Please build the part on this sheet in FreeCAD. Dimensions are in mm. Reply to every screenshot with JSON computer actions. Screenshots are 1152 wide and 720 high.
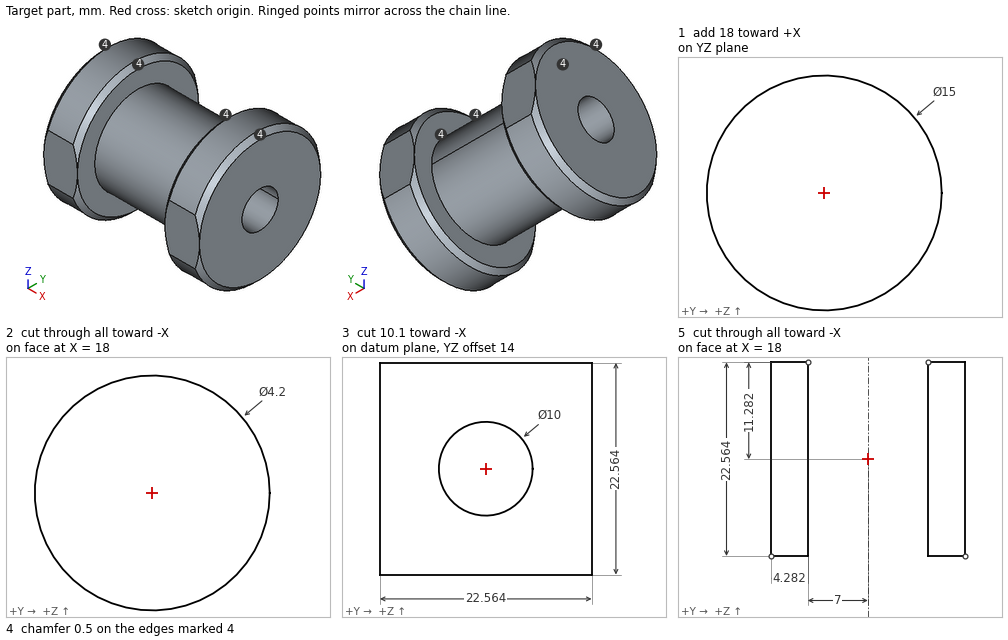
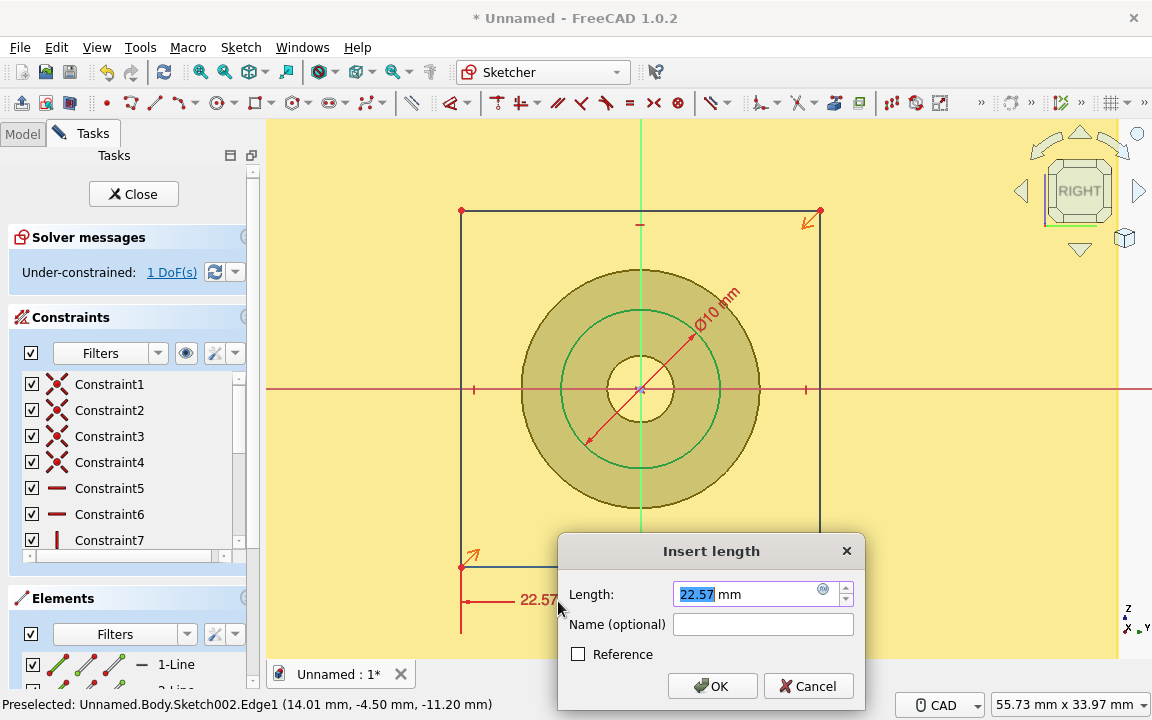
{"action": "type", "text": "22.564"}
{"action": "key", "text": "Return"}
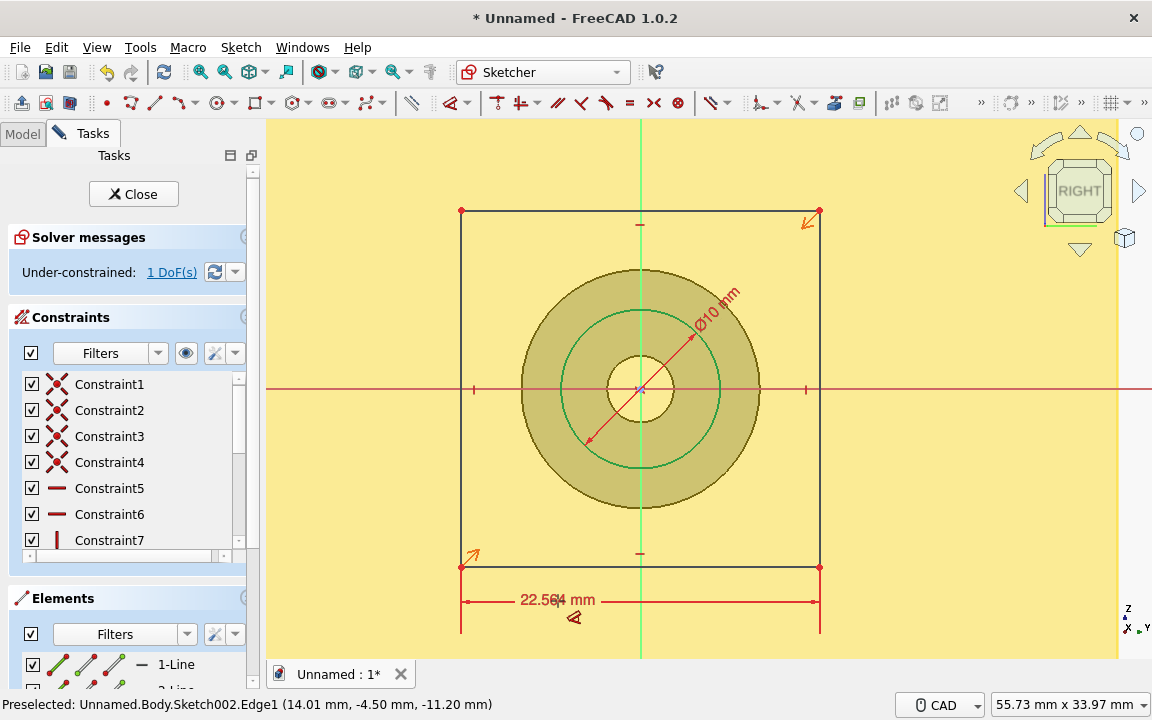
{"action": "left_click", "coordinate": [820, 460]}
{"action": "left_click", "coordinate": [854, 307]}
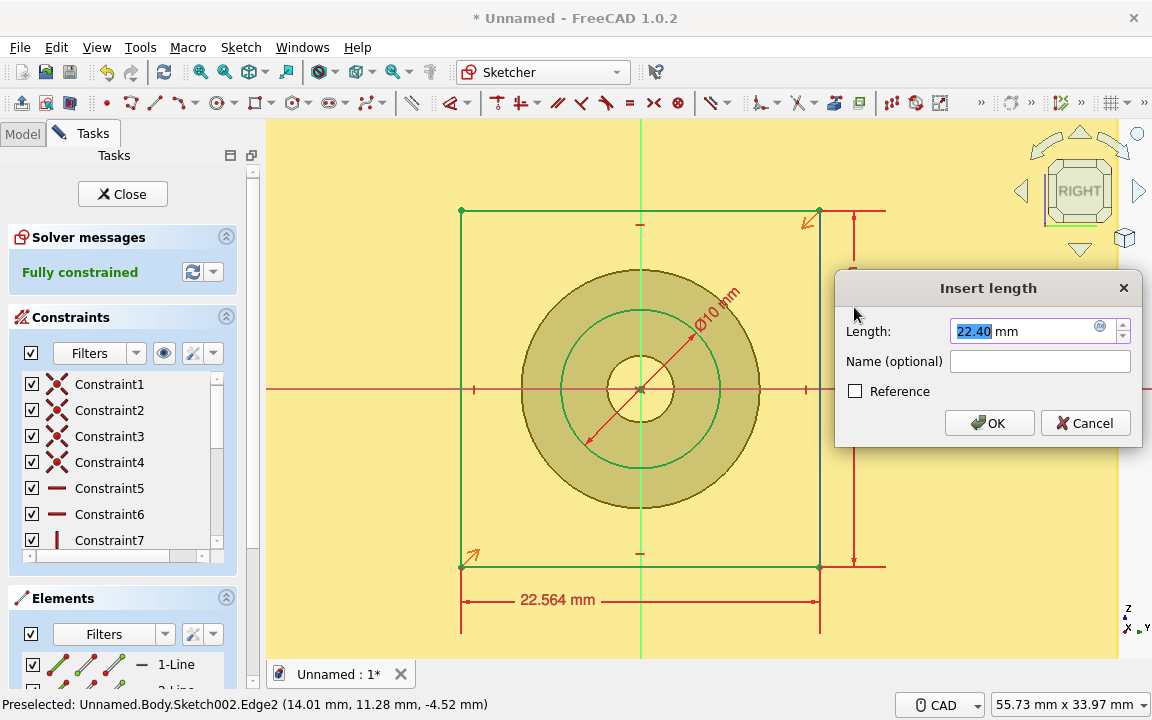
{"action": "type", "text": "22.564"}
{"action": "key", "text": "Return"}
{"action": "key", "text": "Escape"}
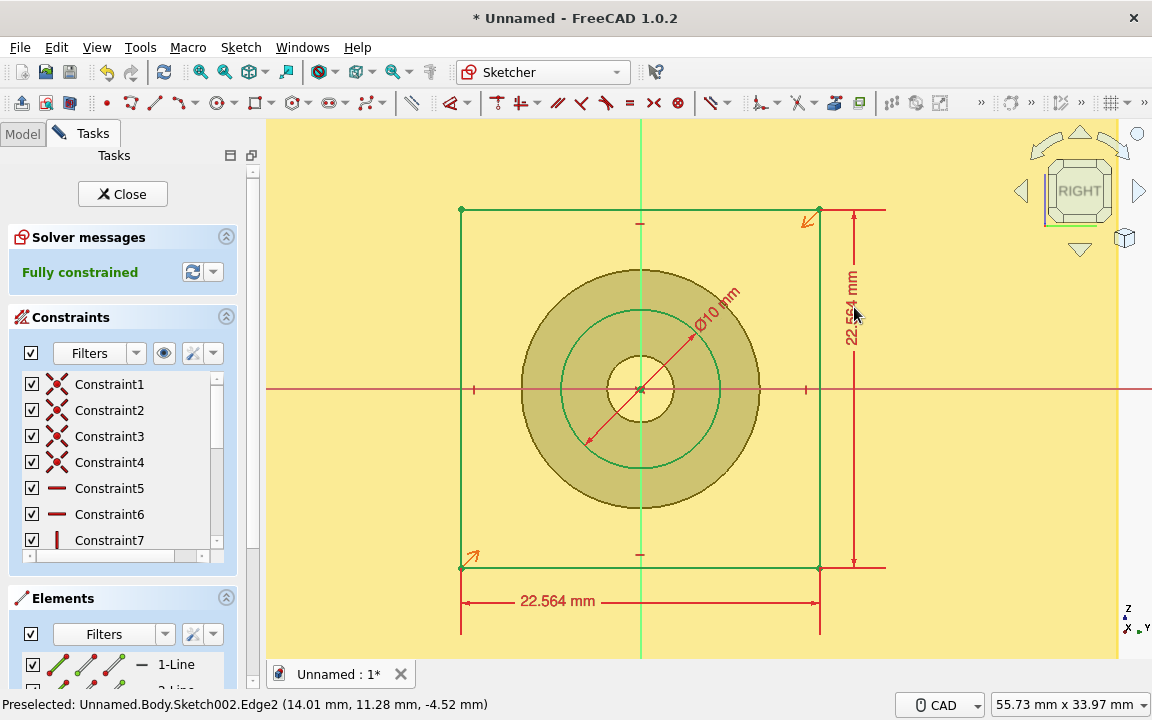
{"action": "left_click", "coordinate": [123, 194]}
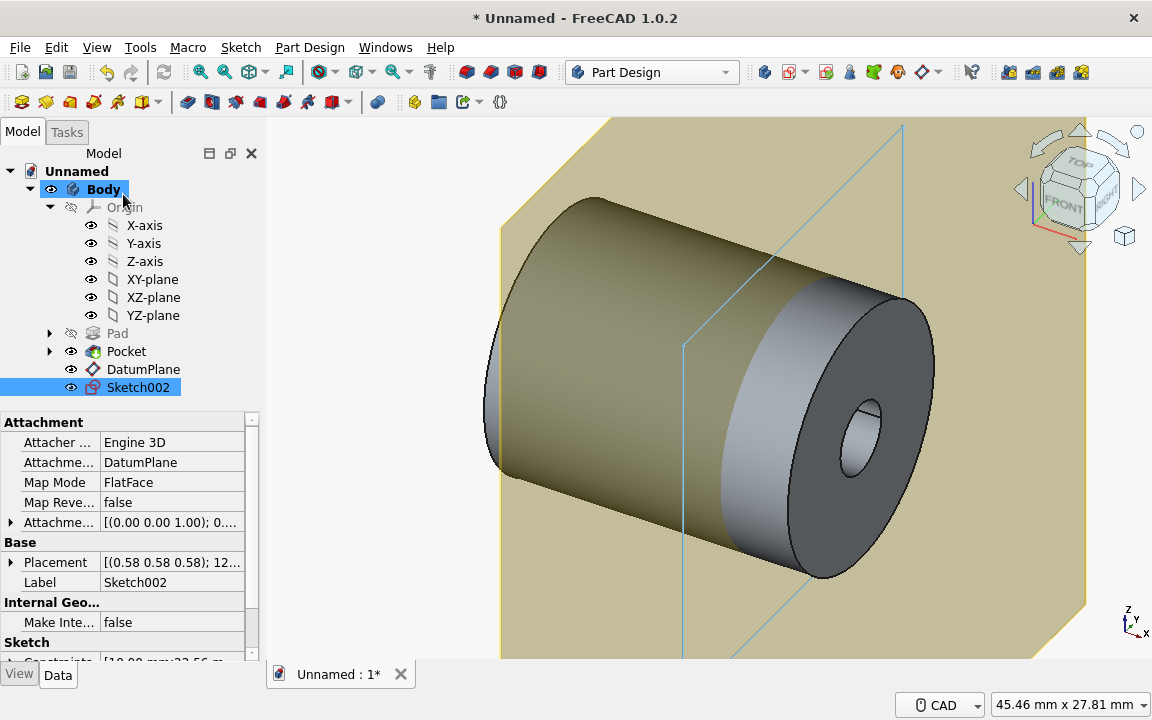
{"action": "left_click", "coordinate": [188, 102]}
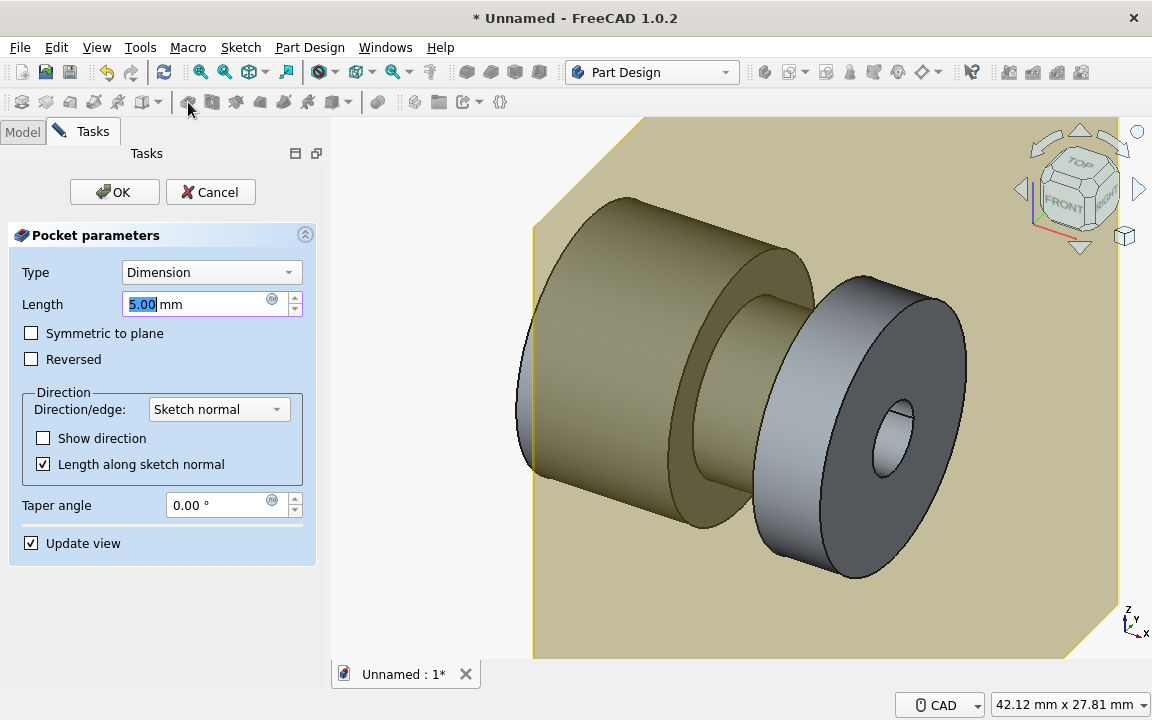
{"action": "type", "text": "10.1"}
{"action": "key", "text": "Tab"}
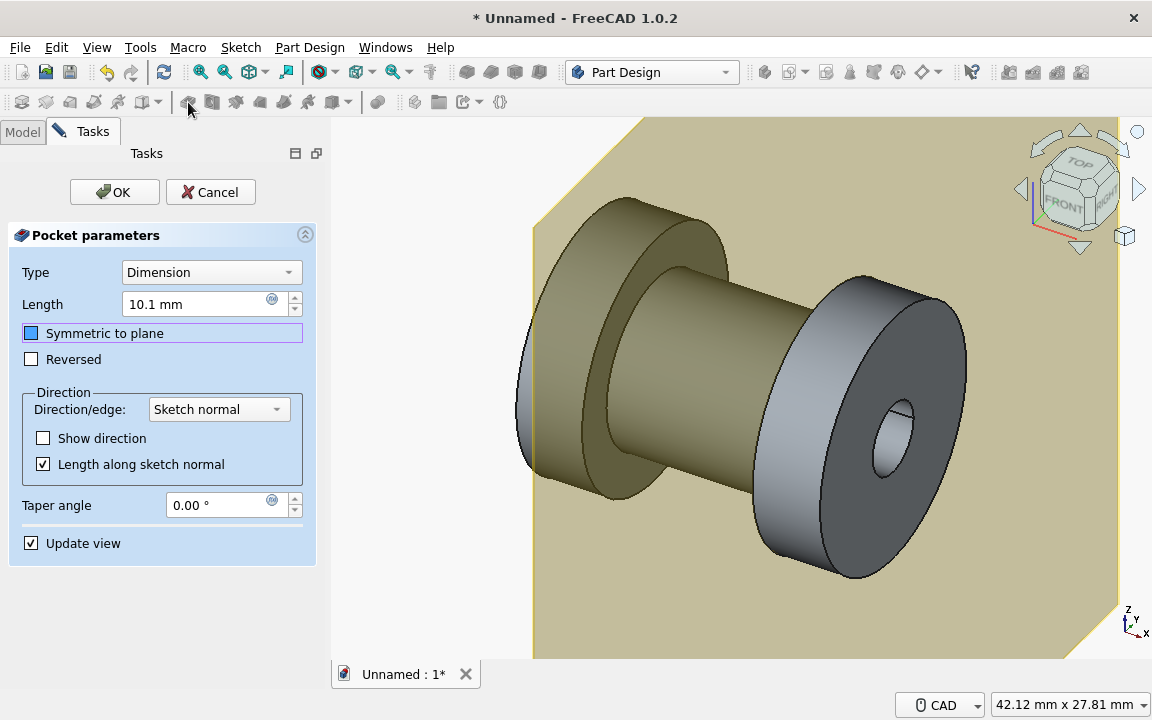
{"action": "left_click", "coordinate": [115, 192]}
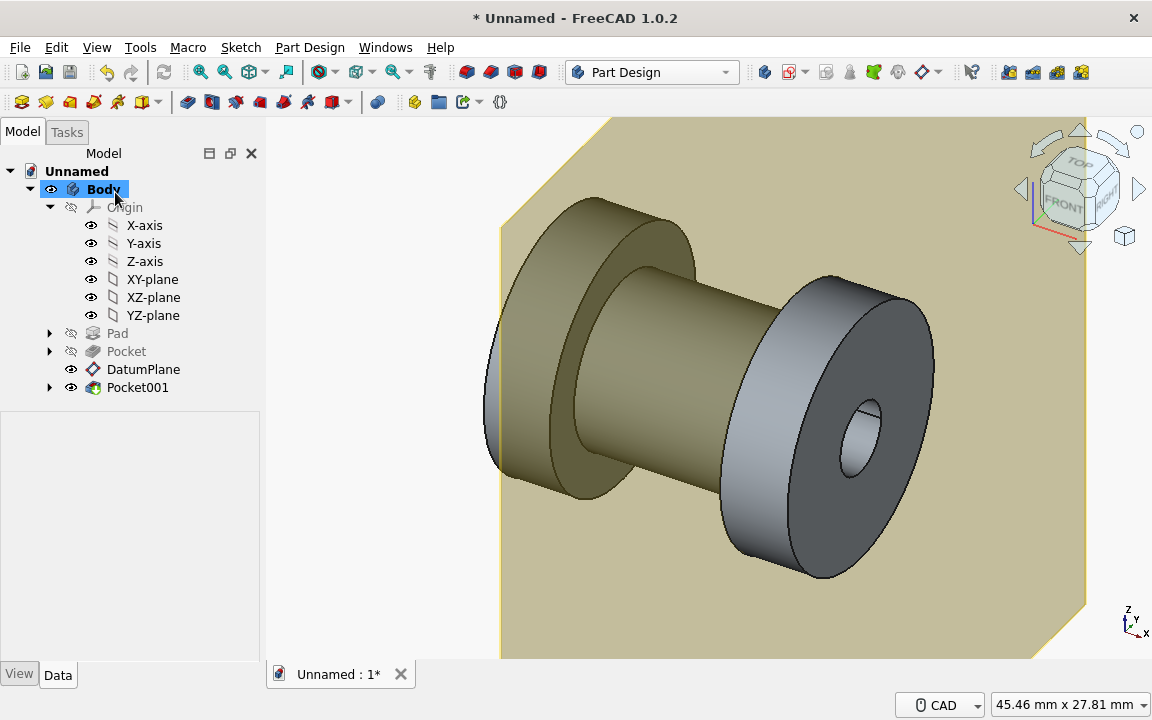
{"action": "left_click", "coordinate": [116, 369]}
{"action": "key", "text": "space"}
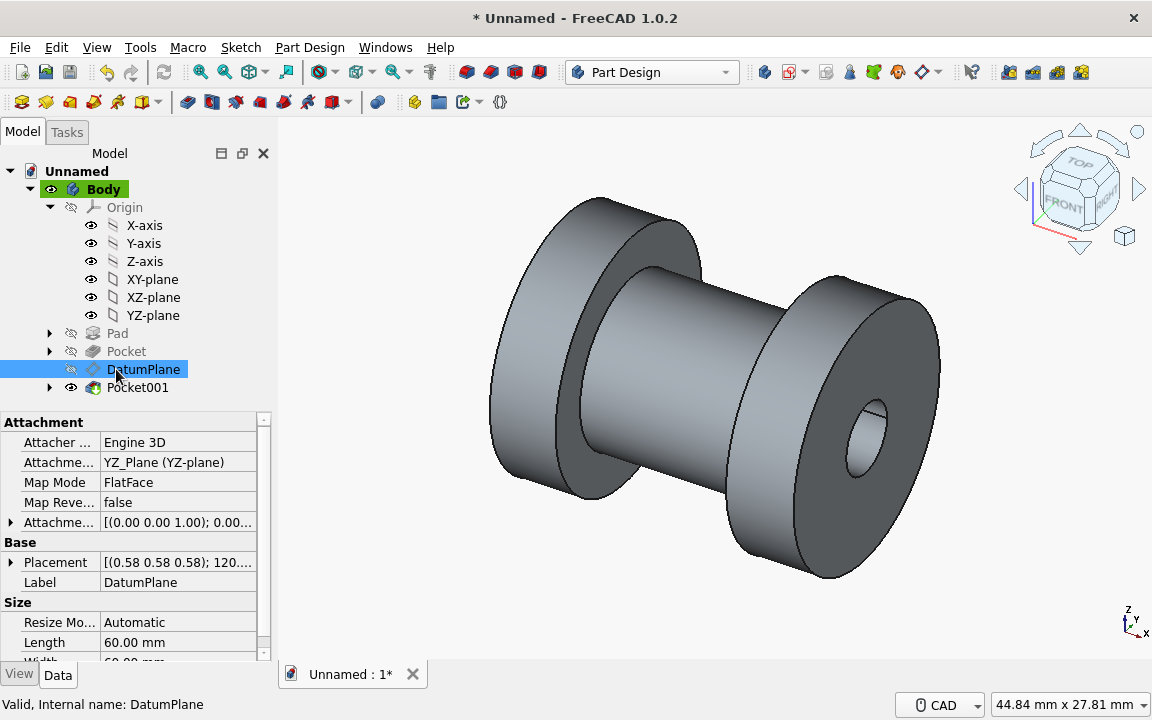
{"action": "left_click", "coordinate": [556, 431]}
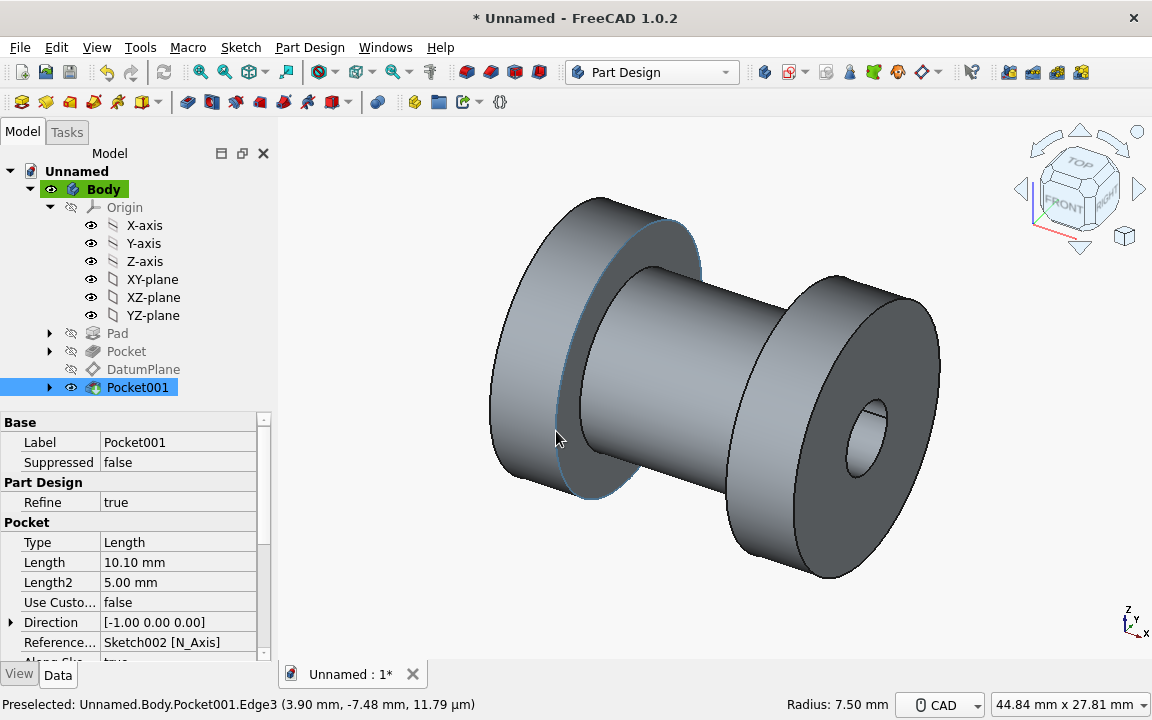
{"action": "left_click", "coordinate": [794, 510], "text": "ctrl"}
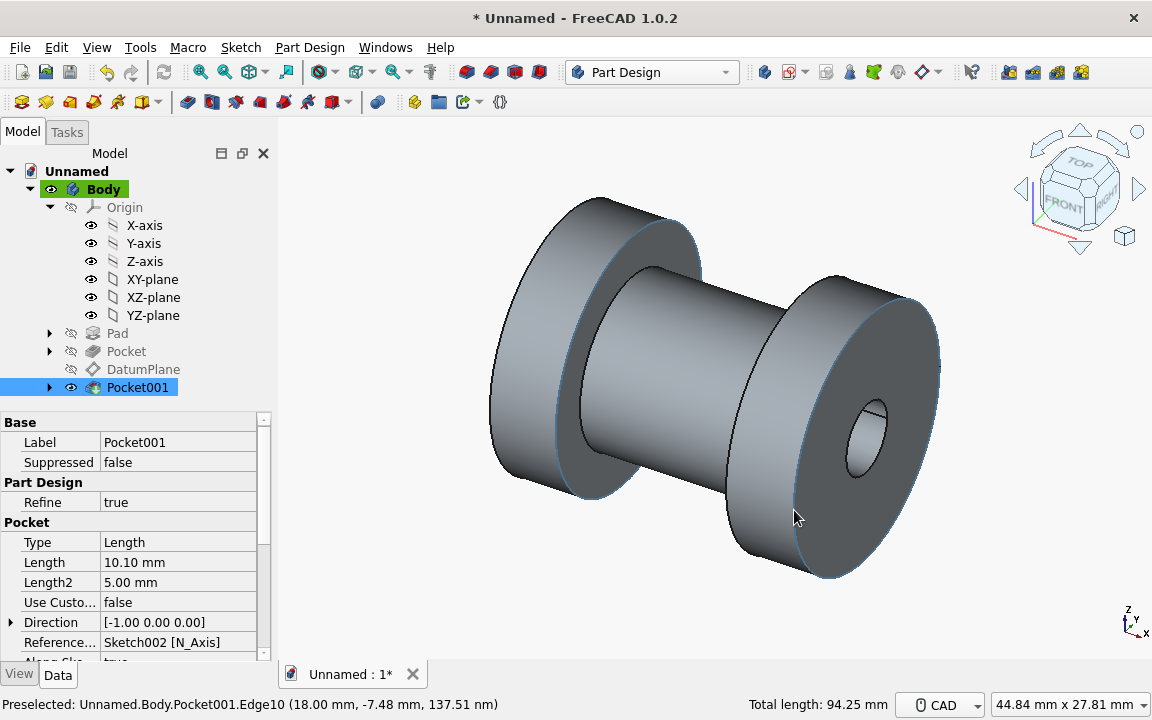
{"action": "key", "text": "0"}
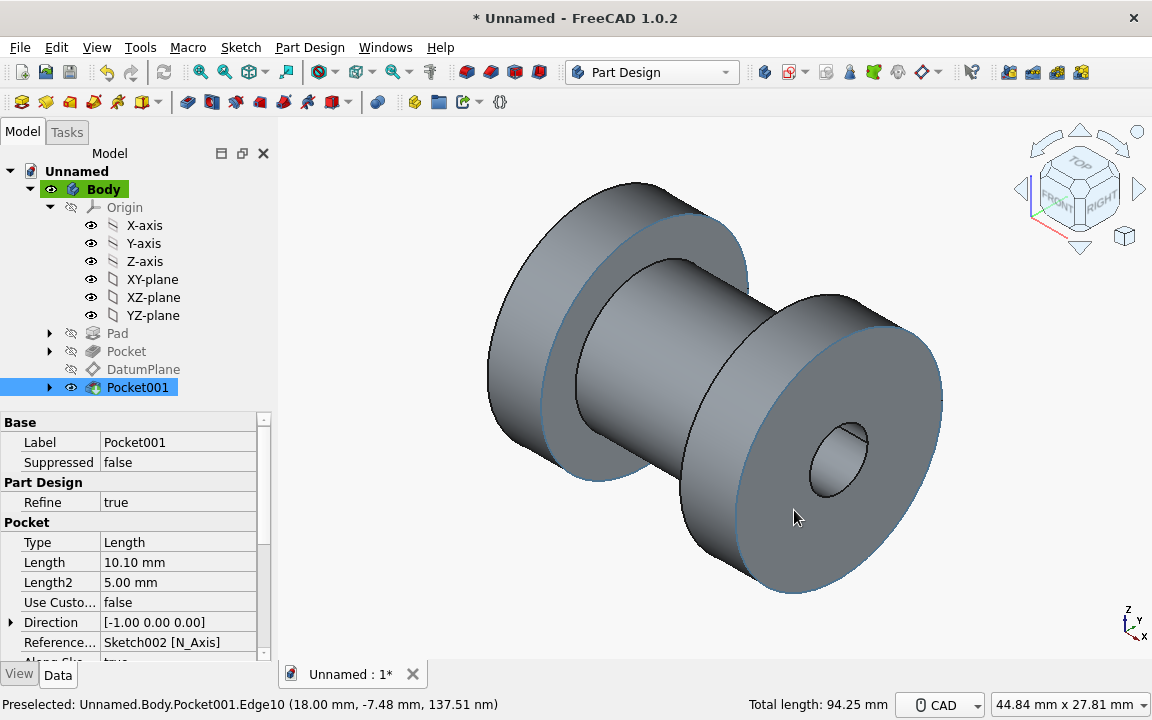
{"action": "key", "text": "2"}